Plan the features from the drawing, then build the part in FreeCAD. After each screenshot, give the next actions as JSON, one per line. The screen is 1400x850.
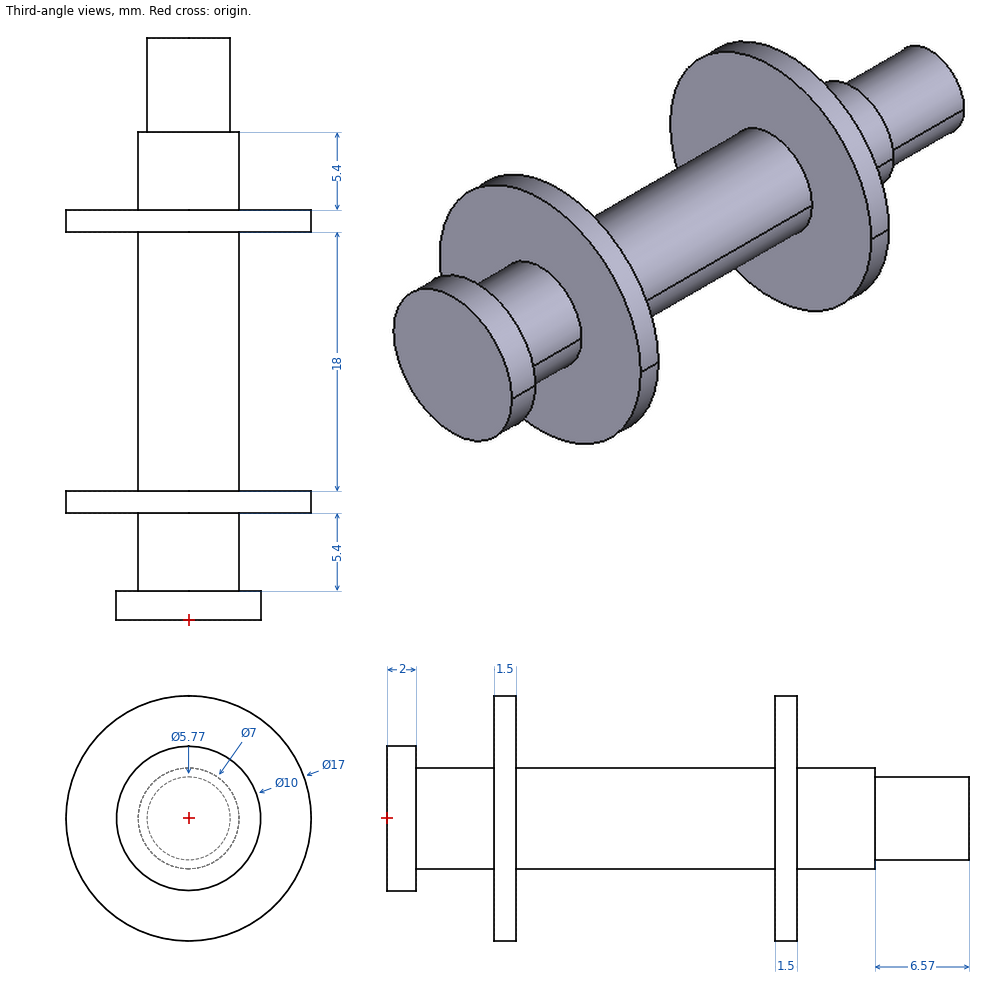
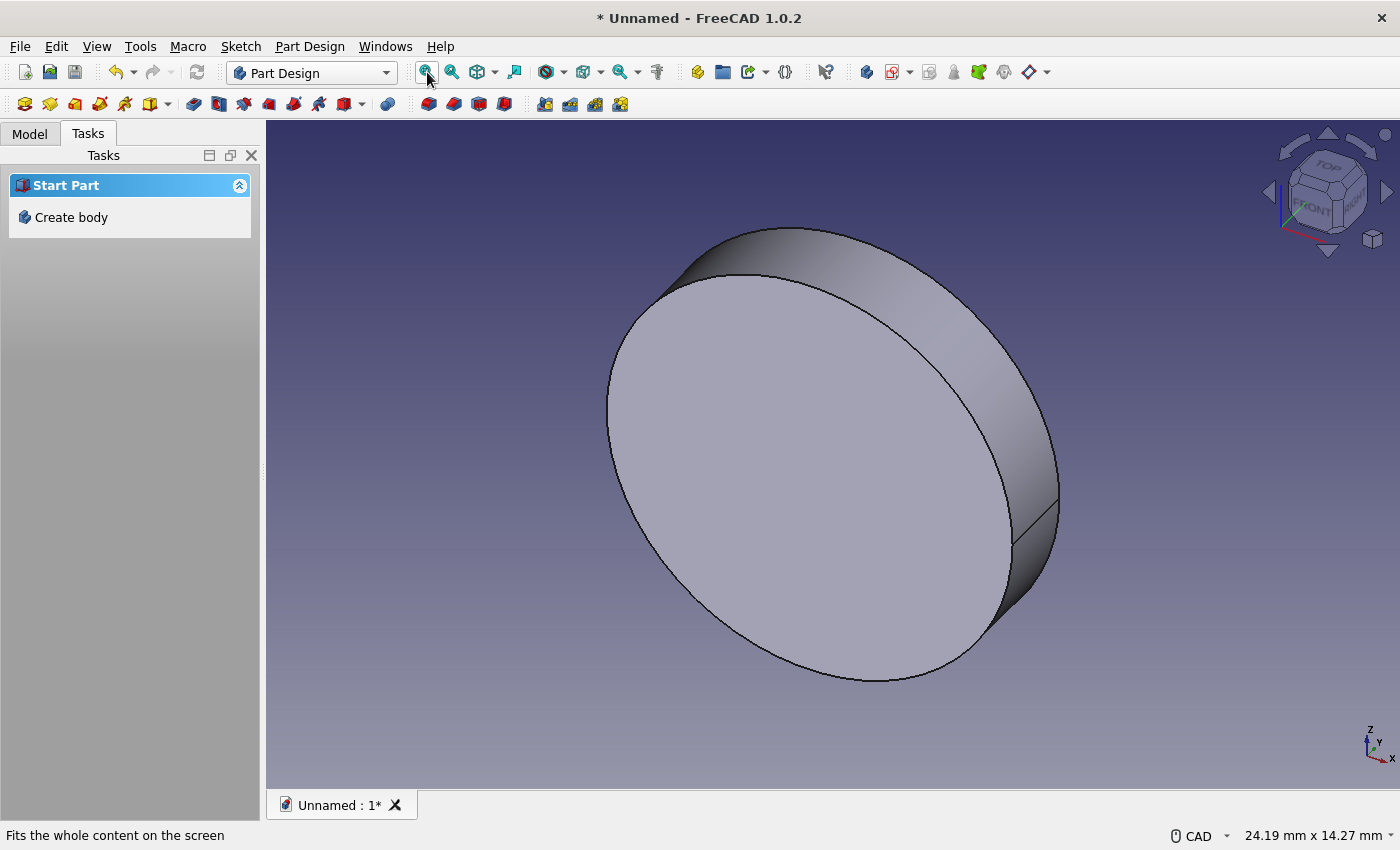
{"action": "key", "text": "4"}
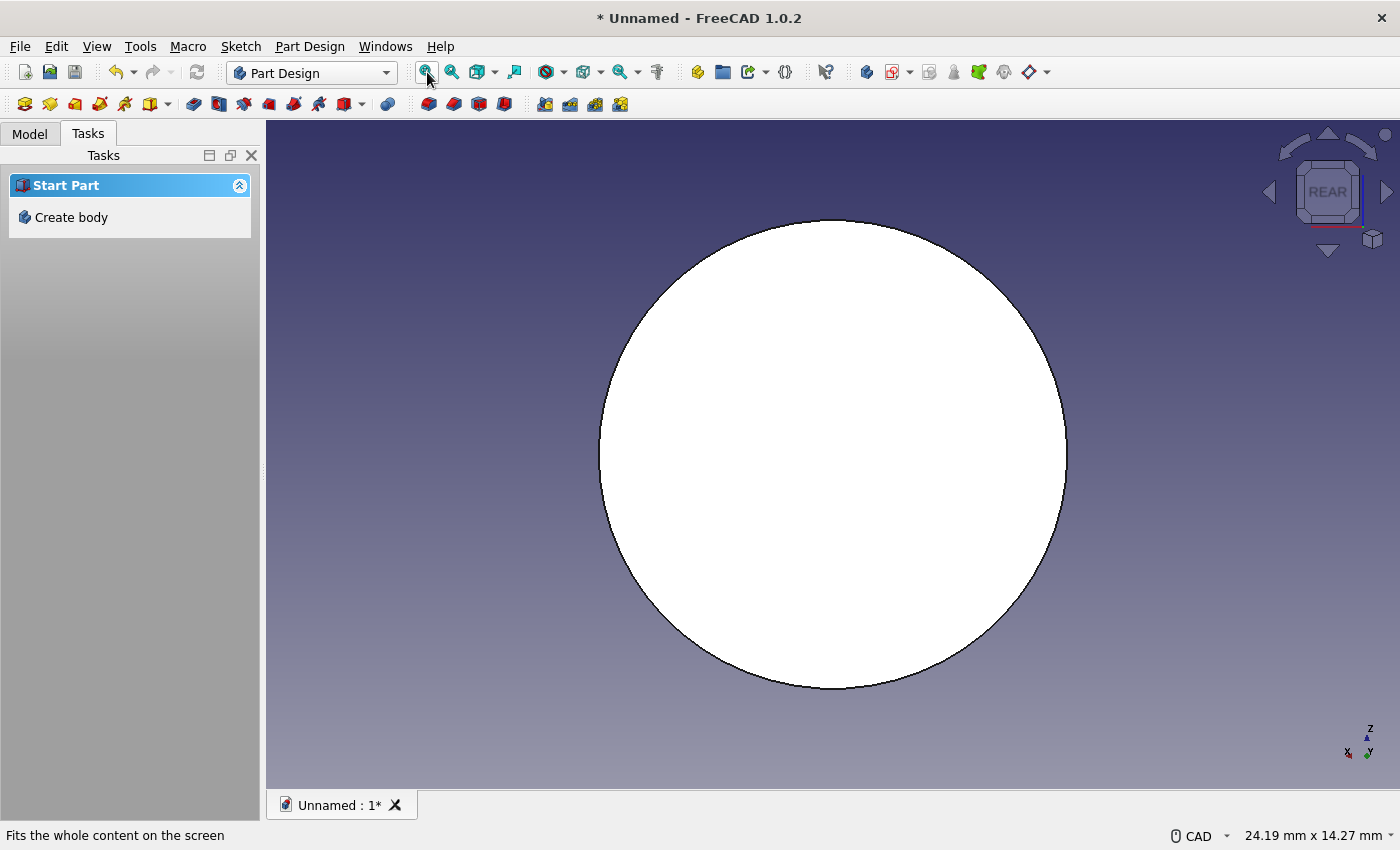
{"action": "left_click", "coordinate": [833, 454]}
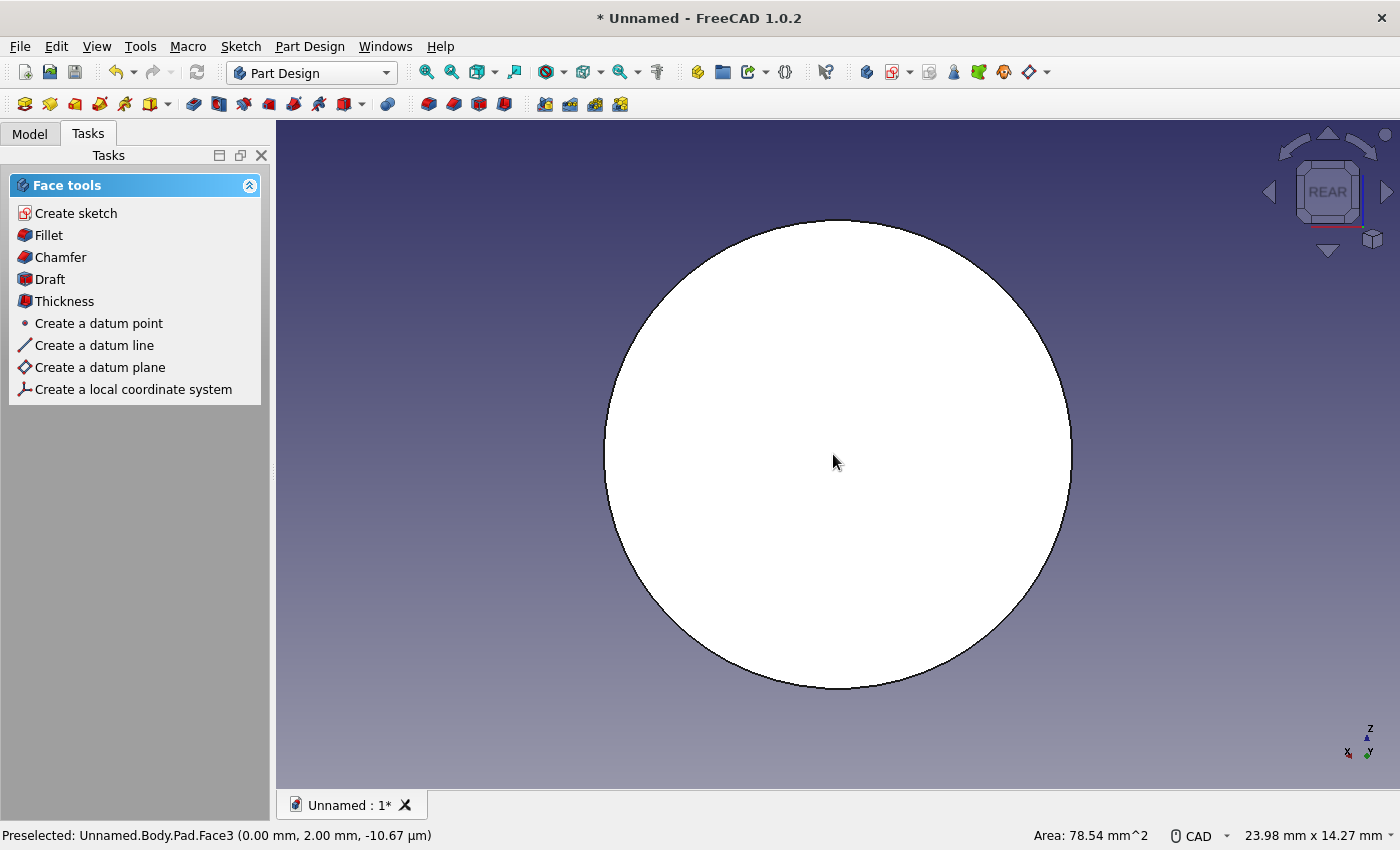
{"action": "left_click", "coordinate": [892, 72]}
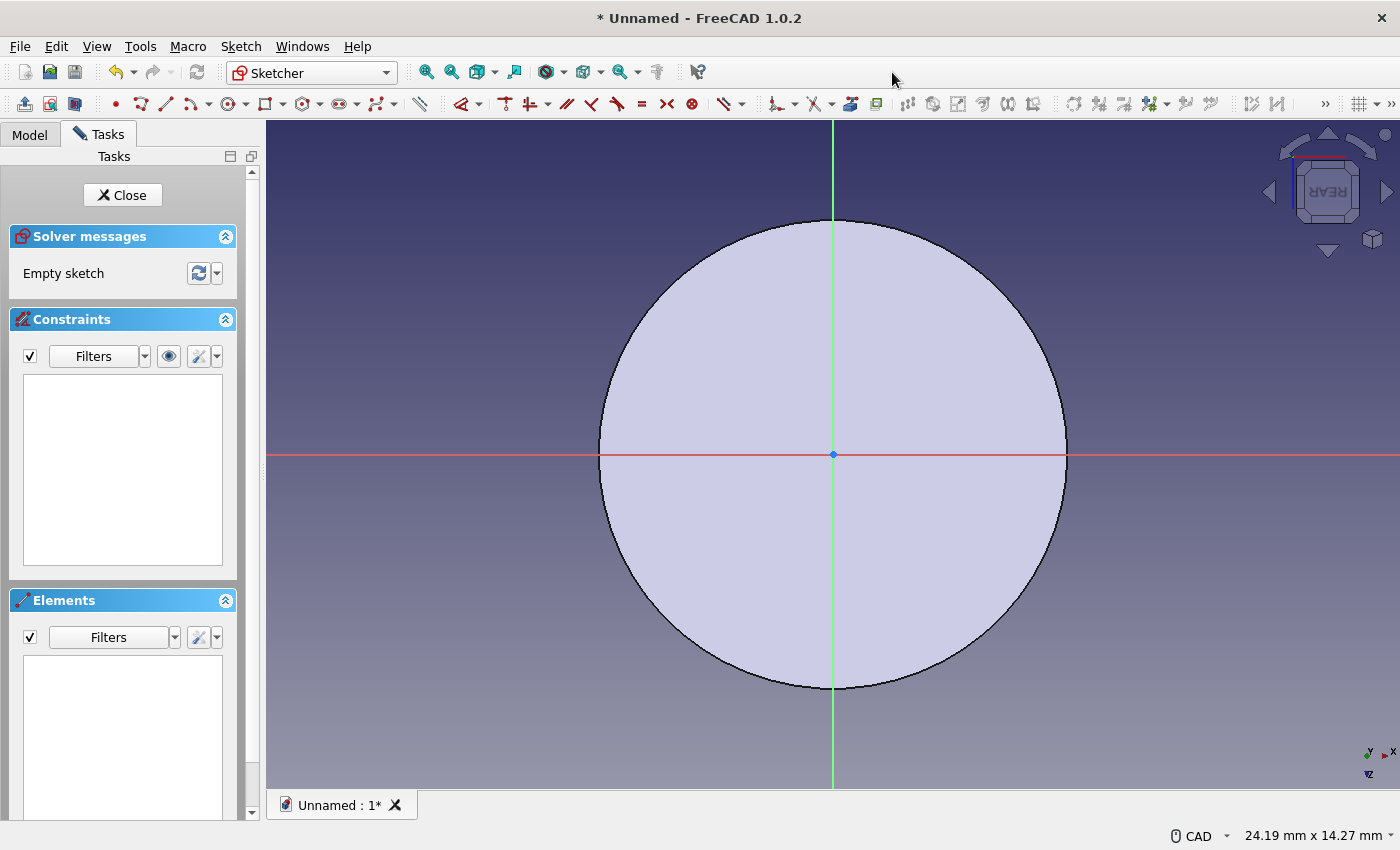
{"action": "left_click", "coordinate": [228, 104]}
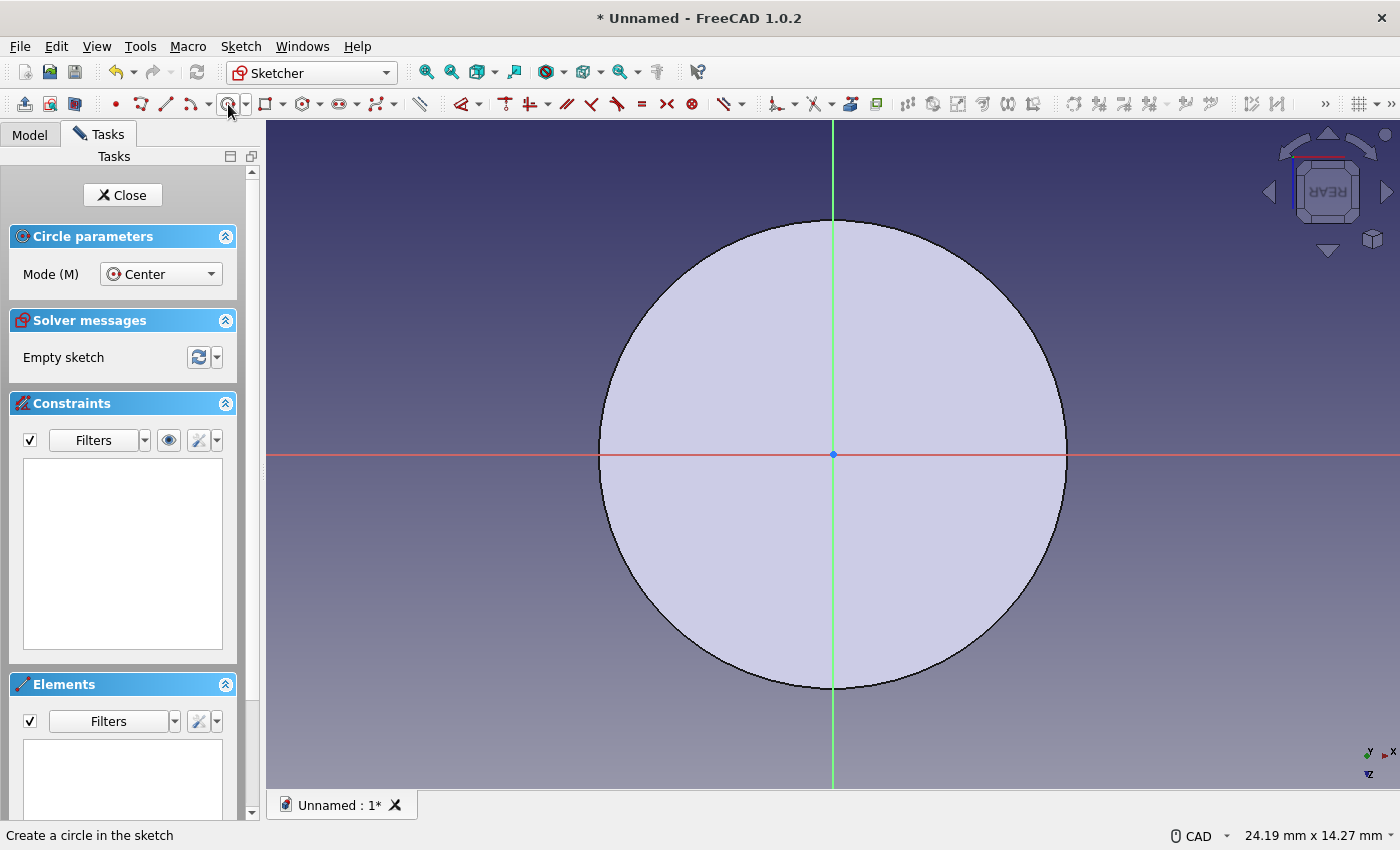
{"action": "left_click", "coordinate": [833, 454]}
{"action": "left_click", "coordinate": [949, 338]}
{"action": "key", "text": "Escape"}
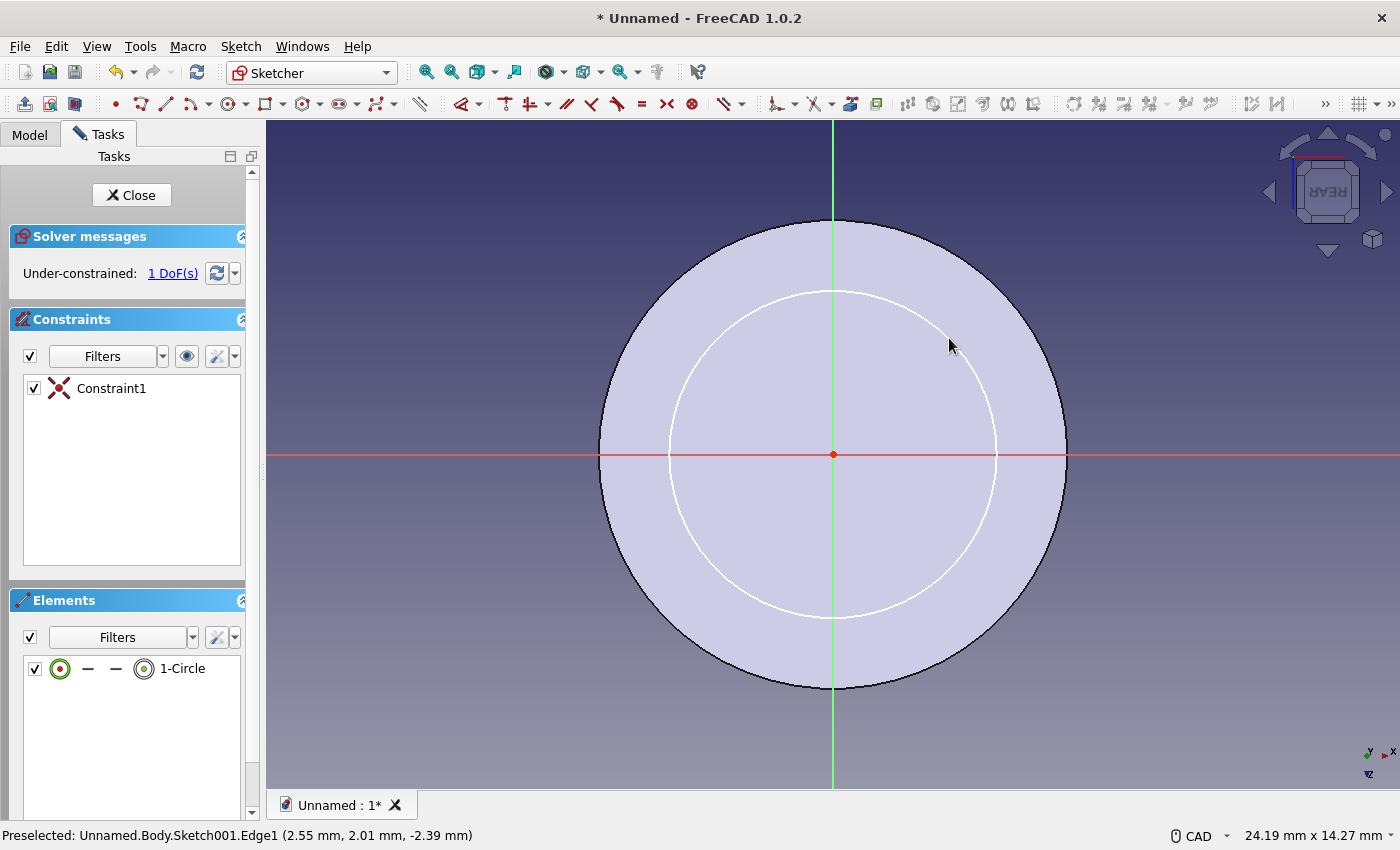
{"action": "left_click", "coordinate": [460, 104]}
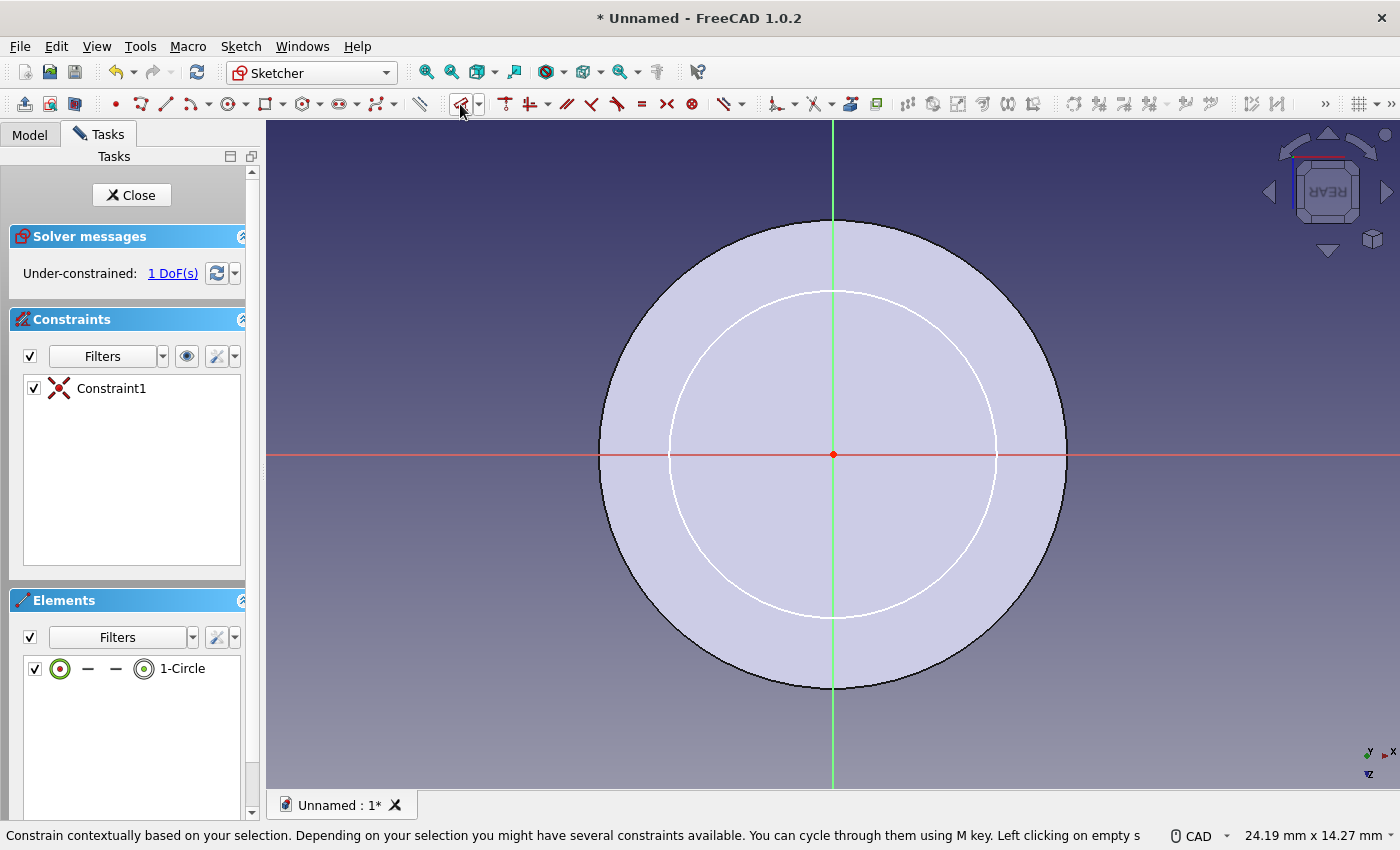
{"action": "left_click", "coordinate": [948, 338]}
{"action": "left_click", "coordinate": [970, 315]}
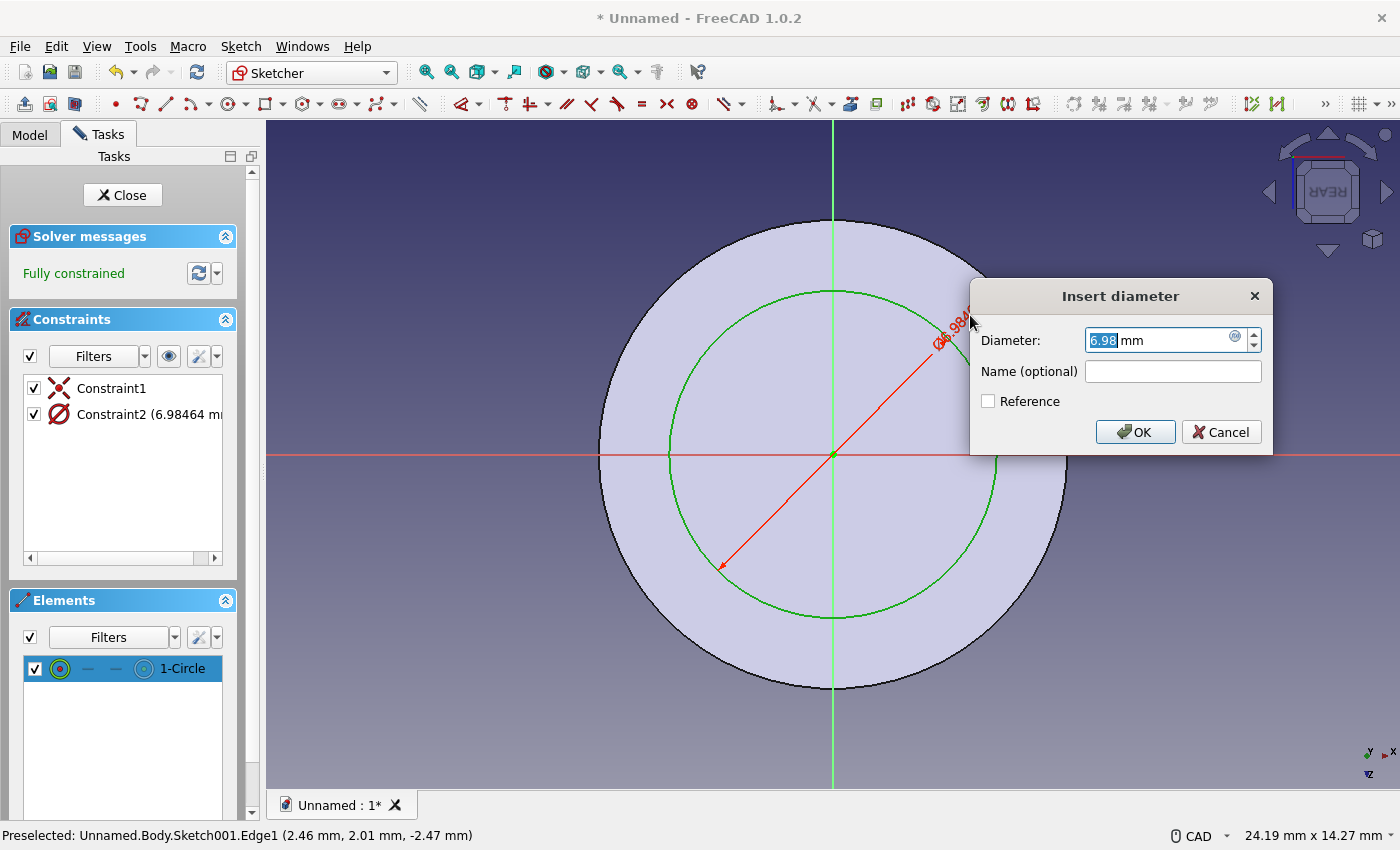
{"action": "type", "text": "7"}
{"action": "key", "text": "Return"}
{"action": "key", "text": "Escape"}